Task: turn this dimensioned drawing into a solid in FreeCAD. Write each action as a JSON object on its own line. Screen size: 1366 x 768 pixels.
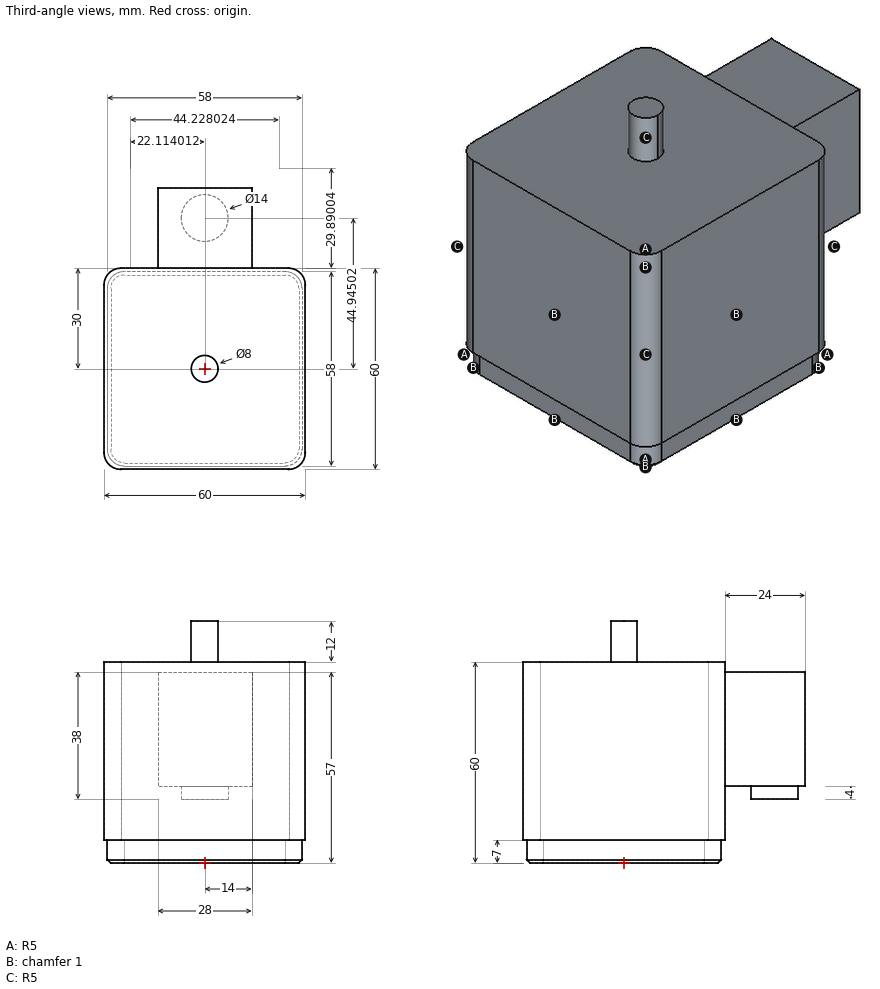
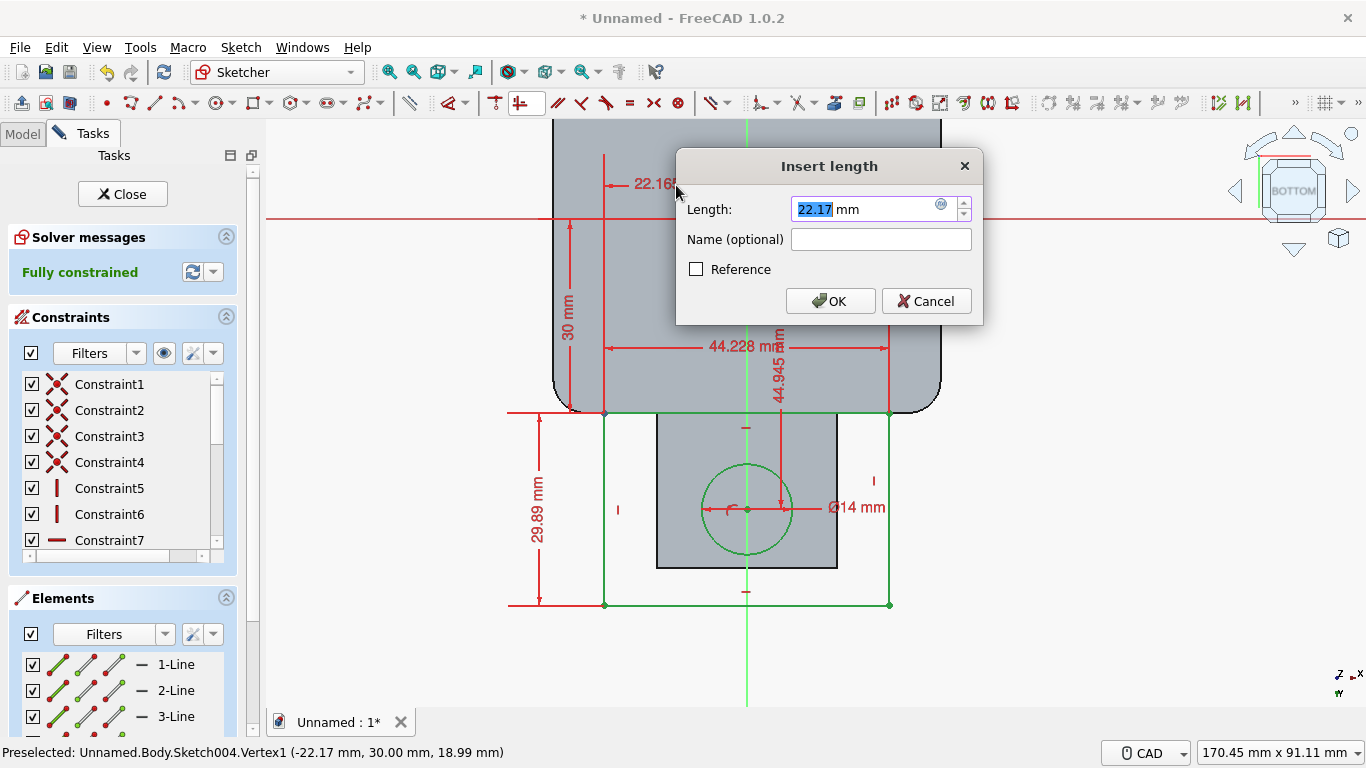
{"action": "type", "text": "22.114012"}
{"action": "key", "text": "Return"}
{"action": "key", "text": "Escape"}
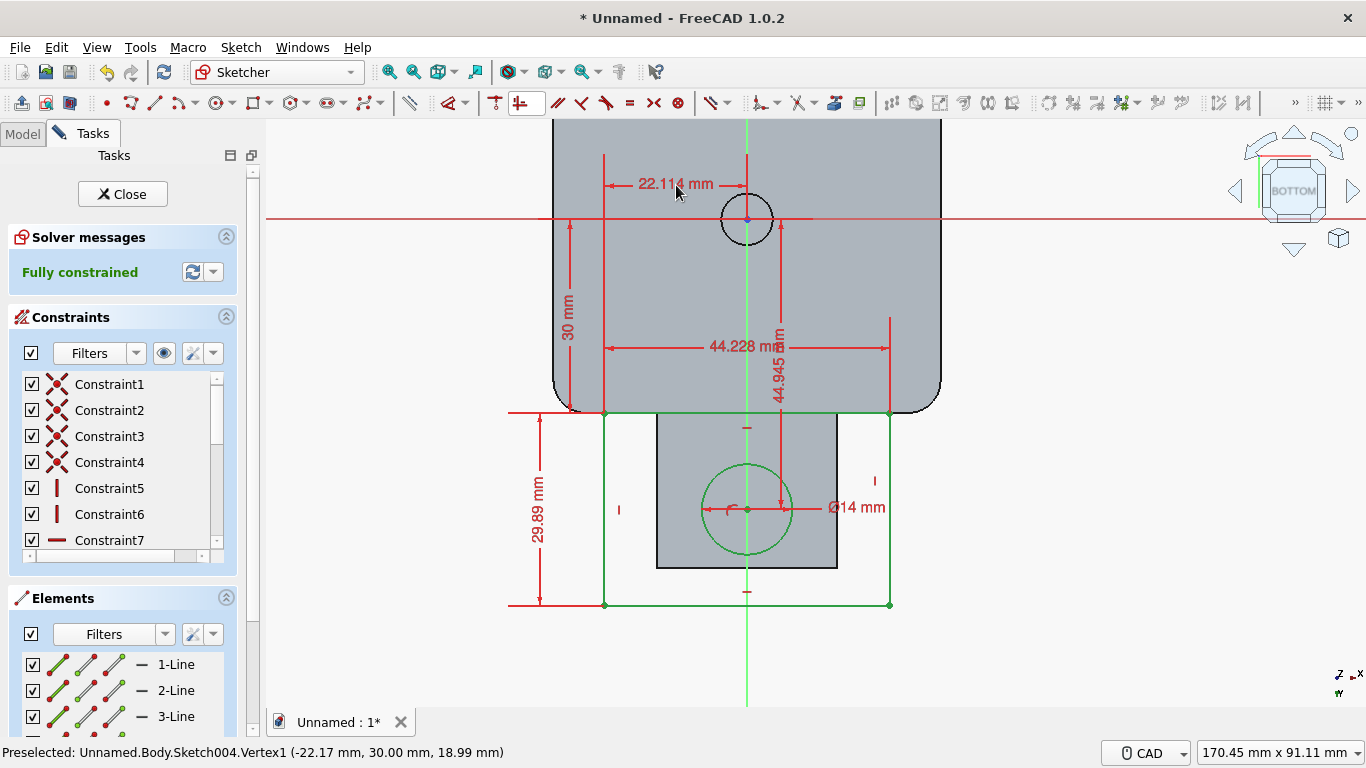
{"action": "left_click", "coordinate": [123, 194]}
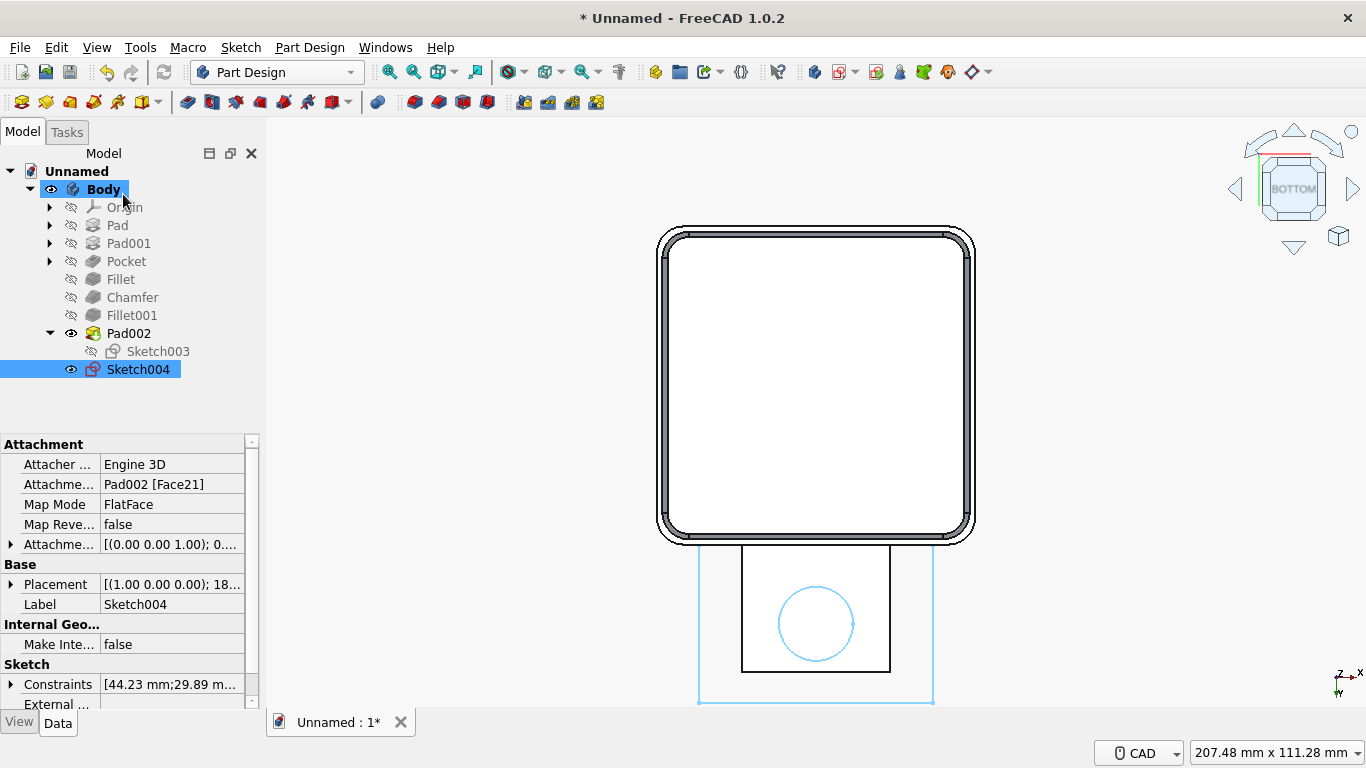
{"action": "left_click", "coordinate": [188, 102]}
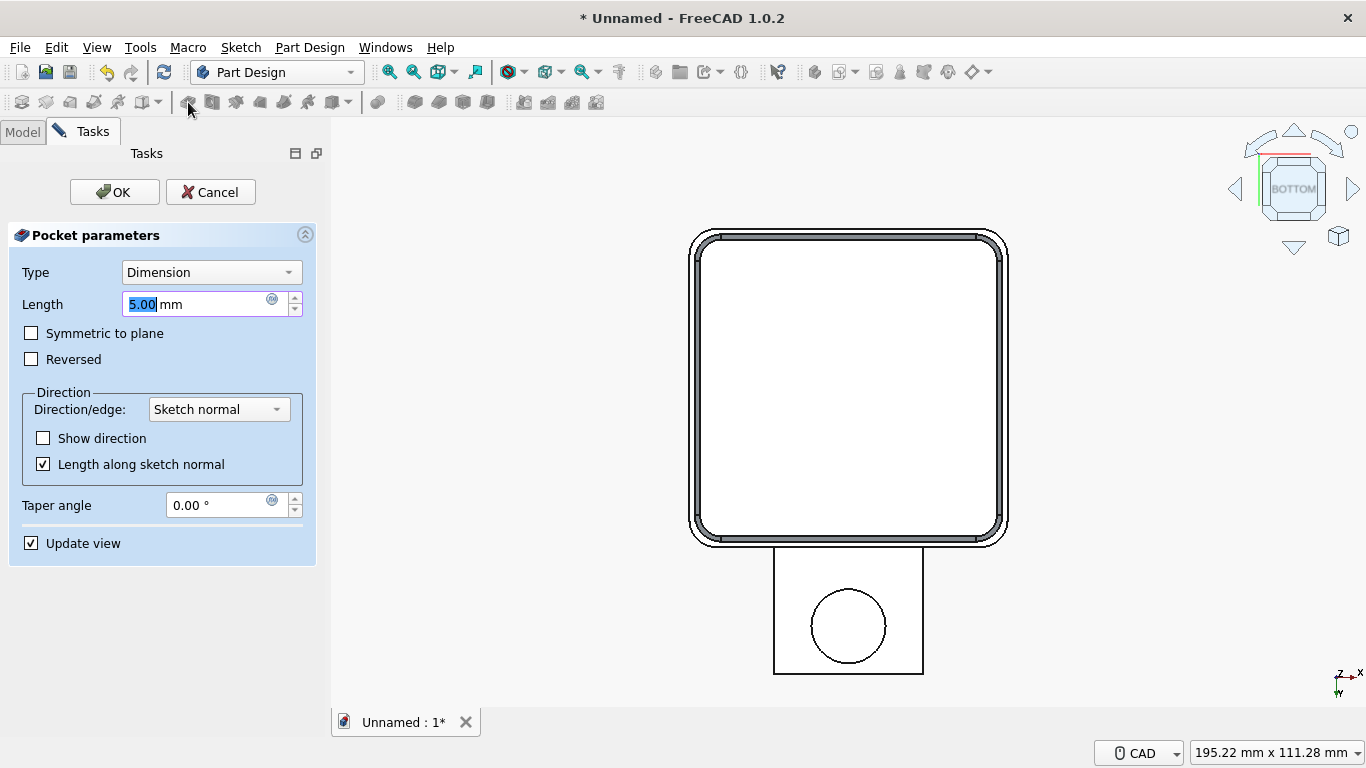
{"action": "type", "text": "4"}
{"action": "key", "text": "Tab"}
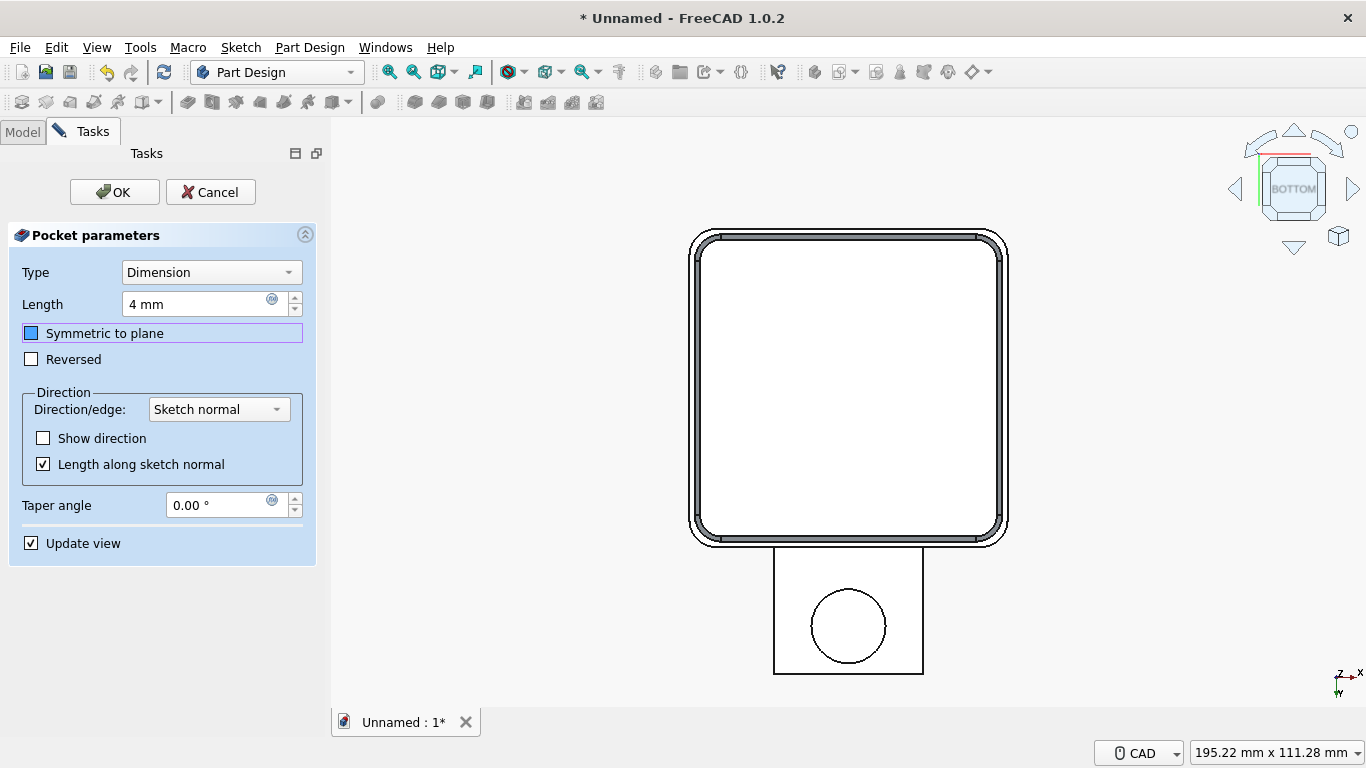
{"action": "left_click", "coordinate": [115, 192]}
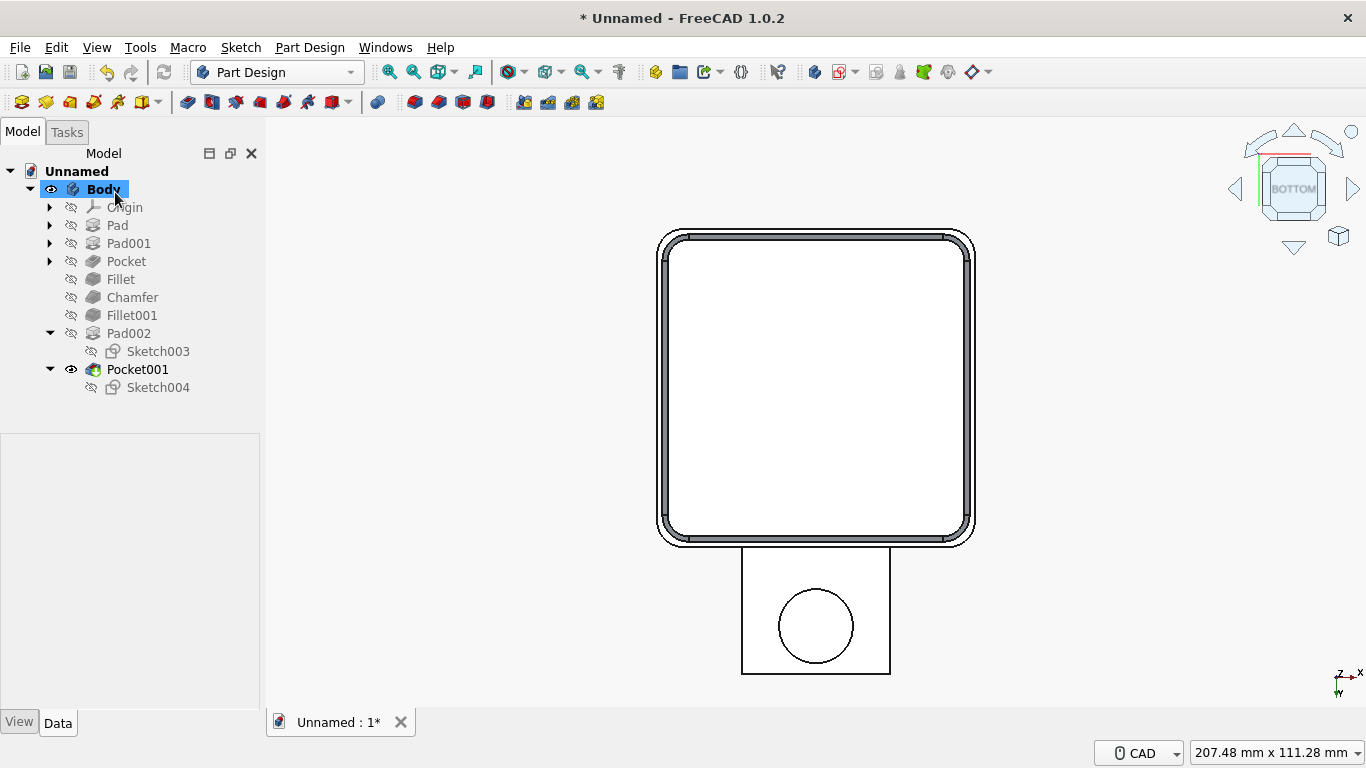
{"action": "key", "text": "0"}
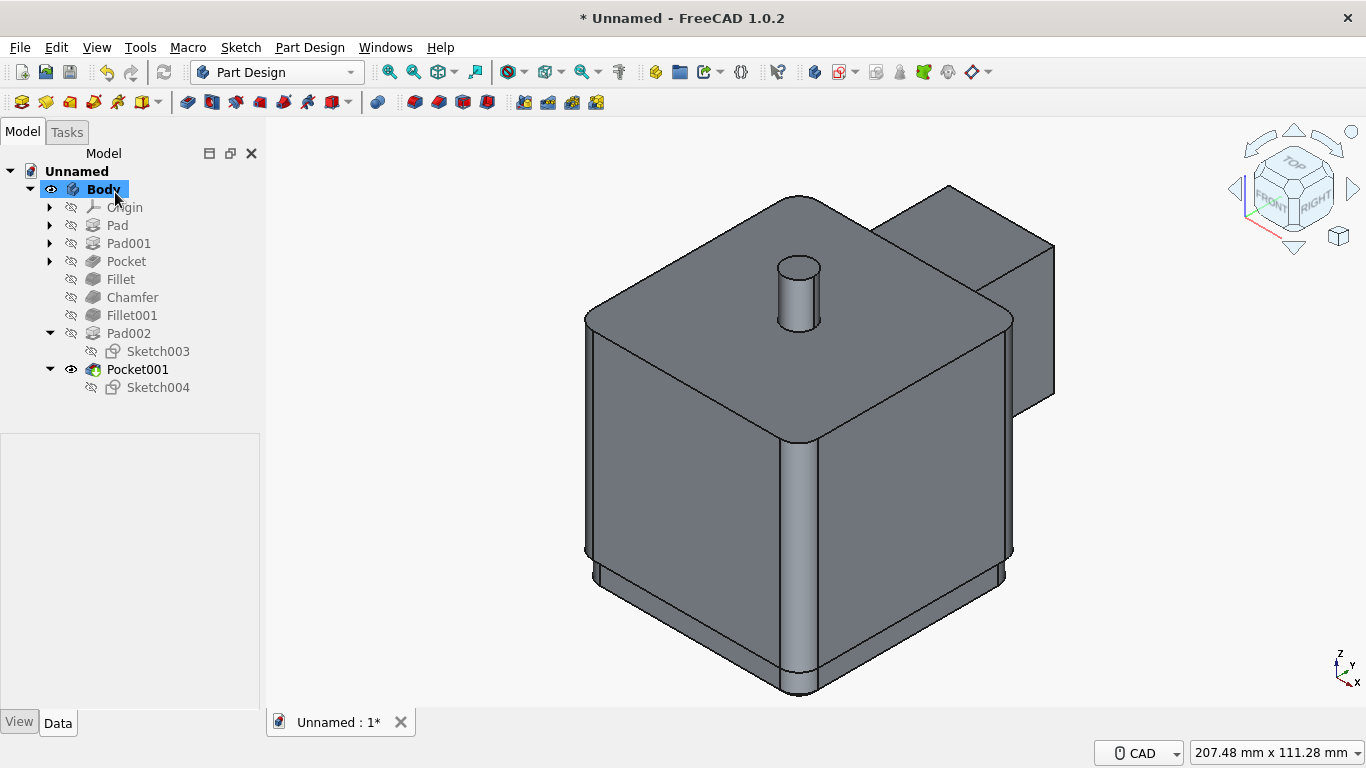
{"action": "left_click", "coordinate": [390, 72]}